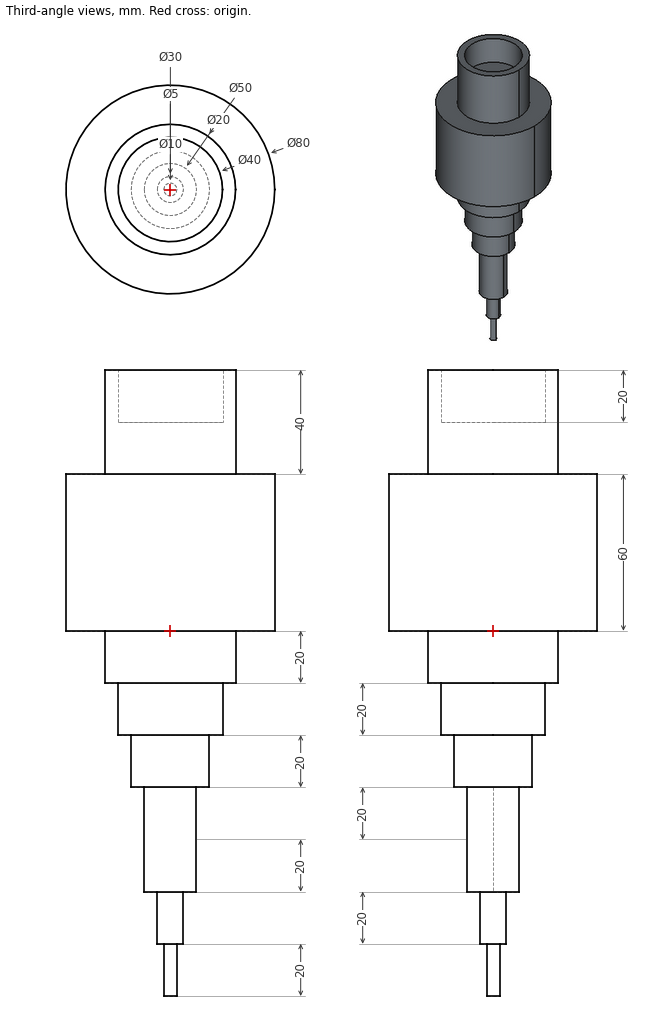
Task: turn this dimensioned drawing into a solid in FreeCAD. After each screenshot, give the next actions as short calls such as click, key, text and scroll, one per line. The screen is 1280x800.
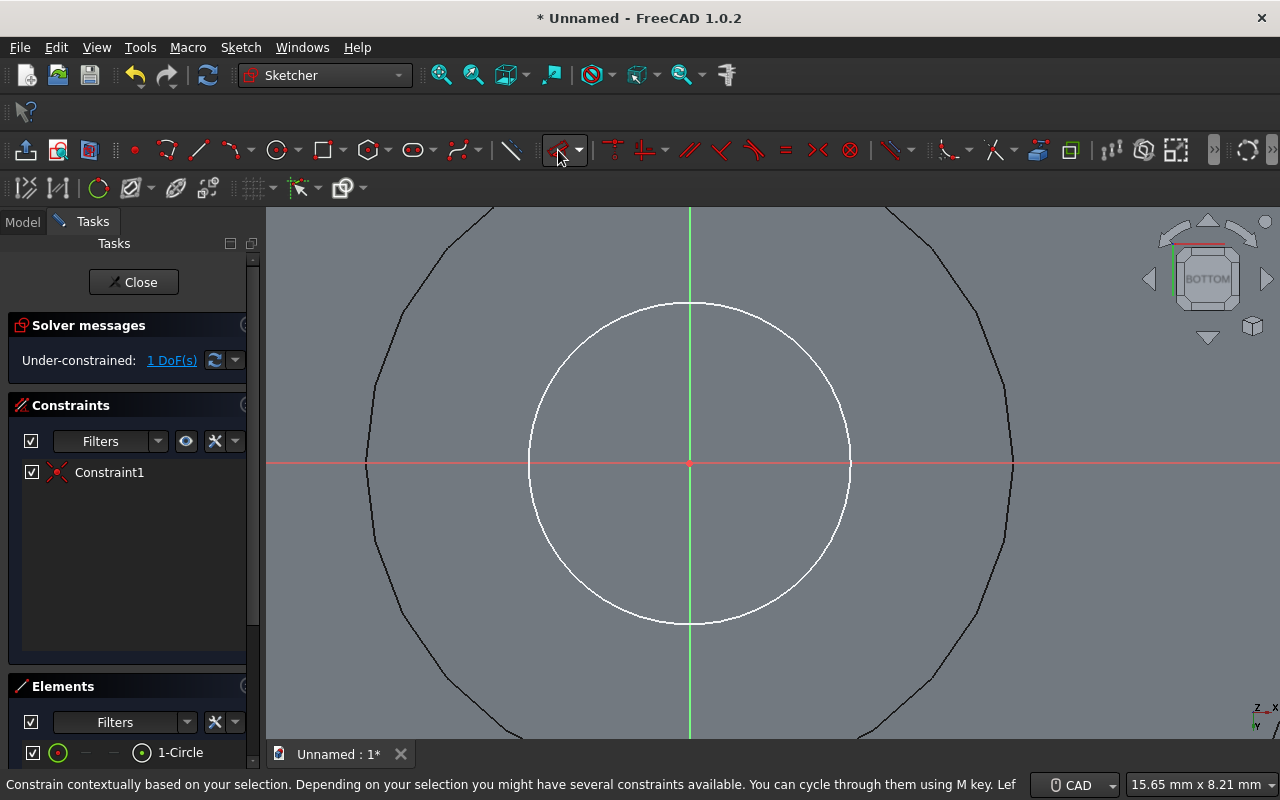
click(803, 349)
click(826, 326)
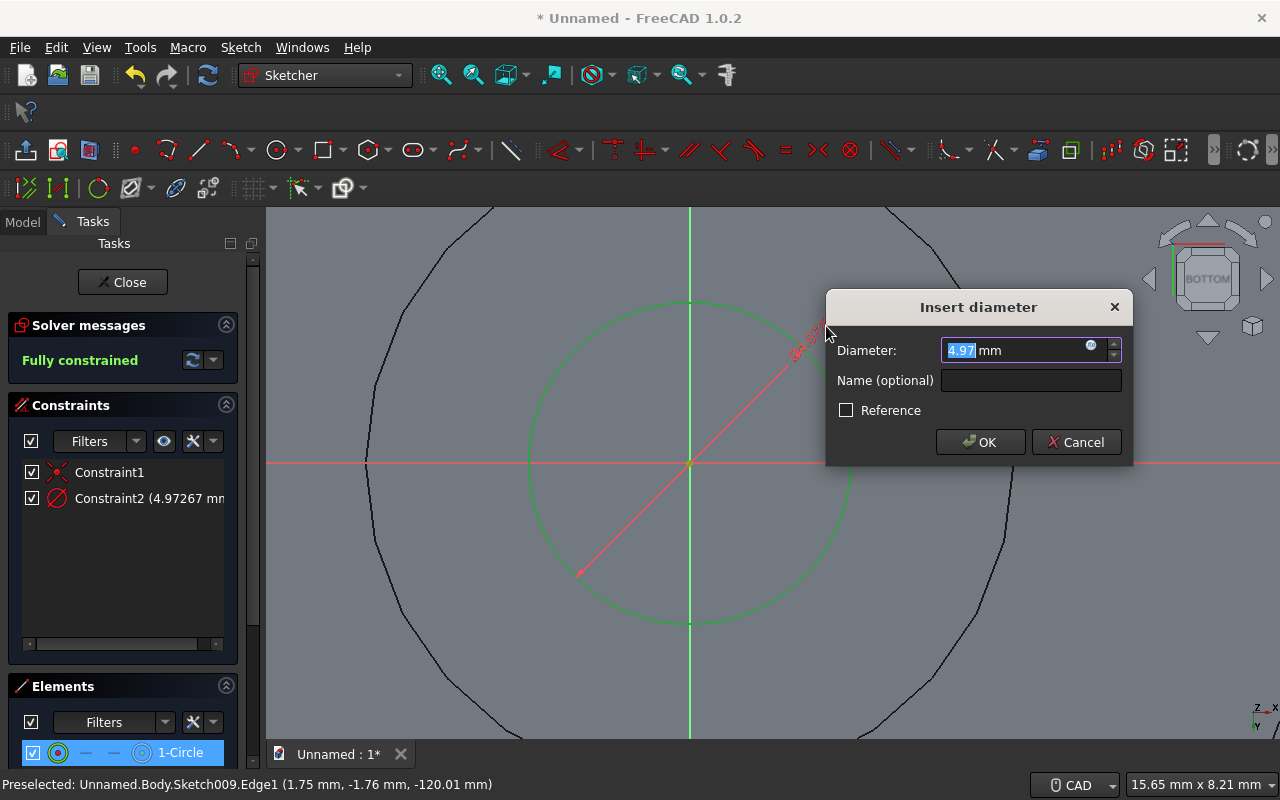
text(5)
key(Return)
key(Escape)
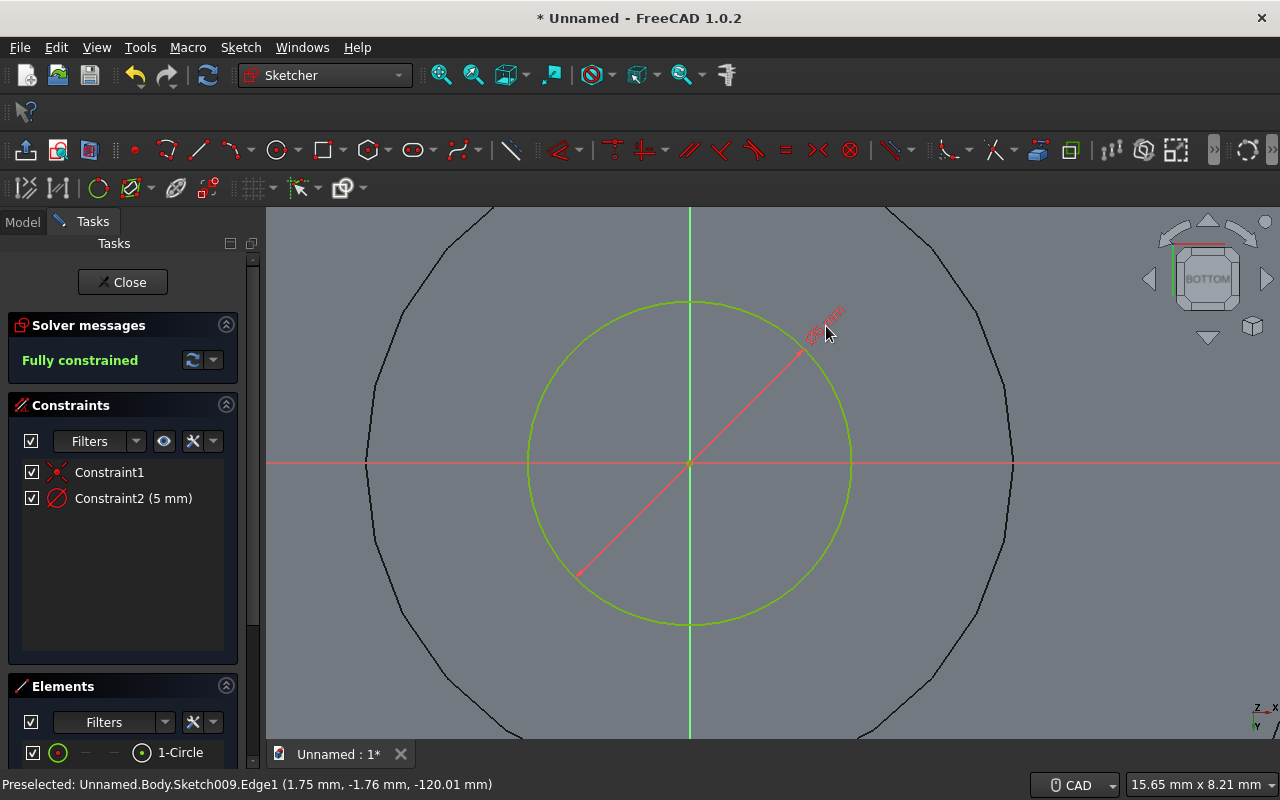
click(123, 282)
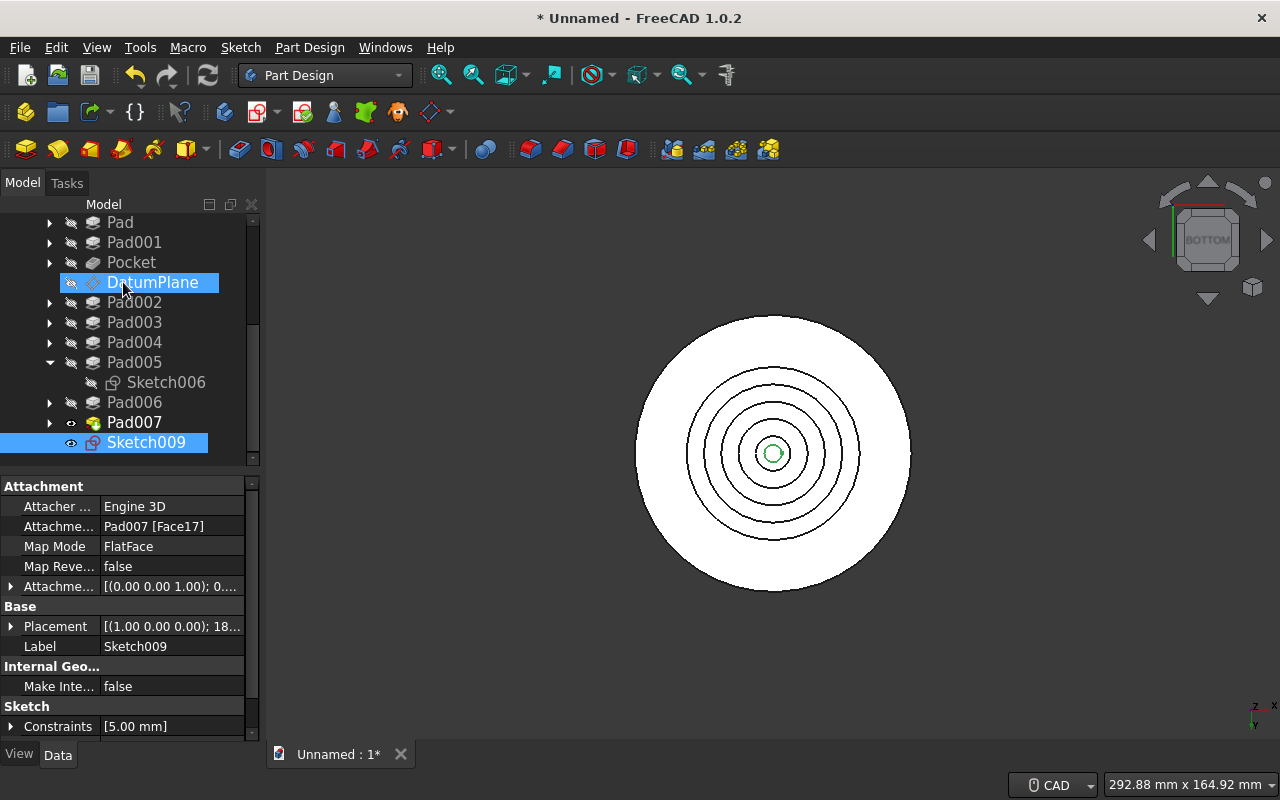
click(26, 150)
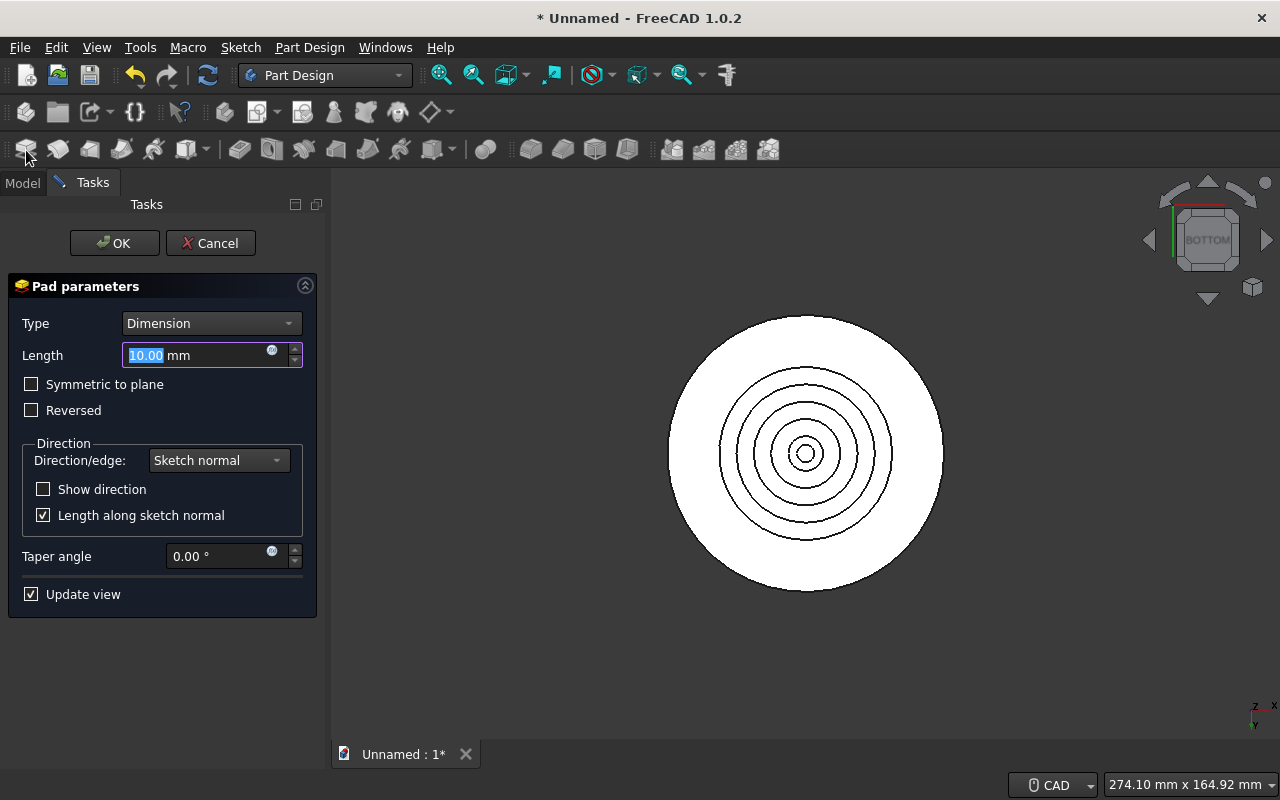
text(20)
key(Tab)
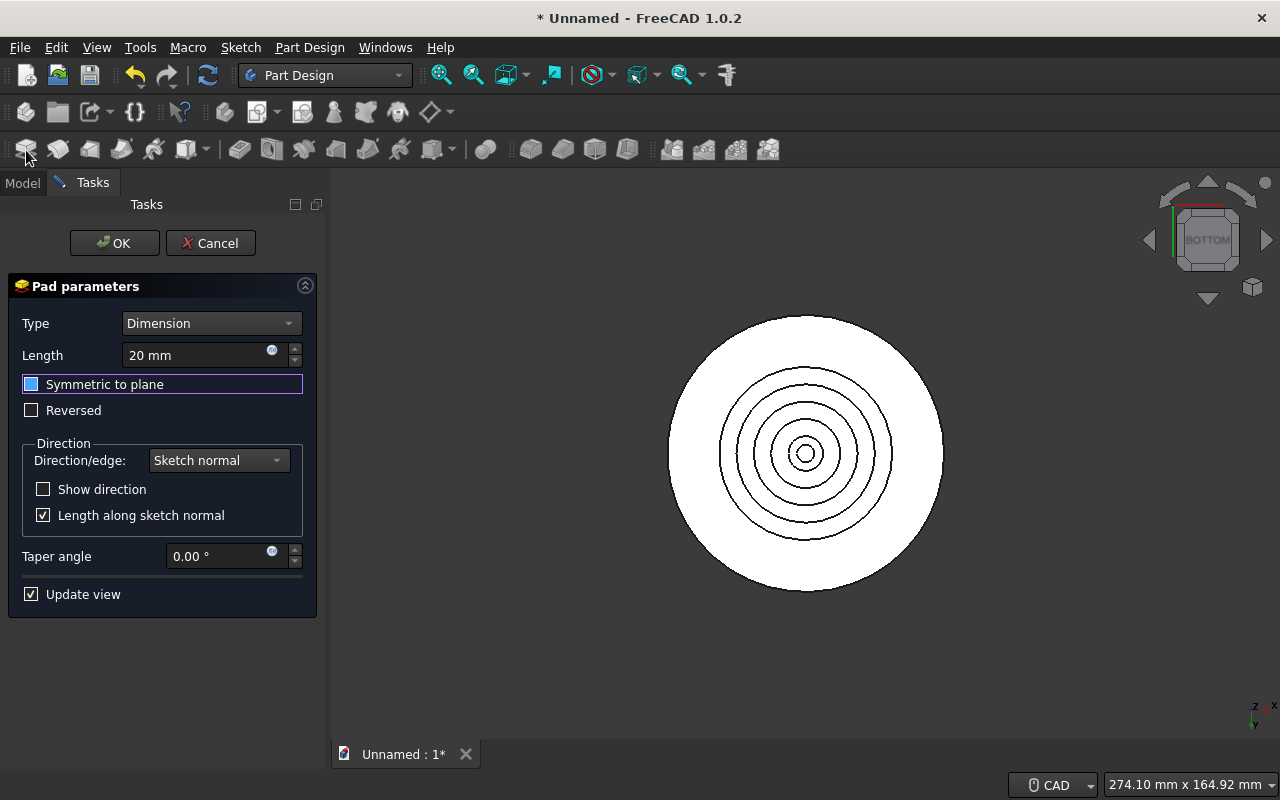
click(115, 243)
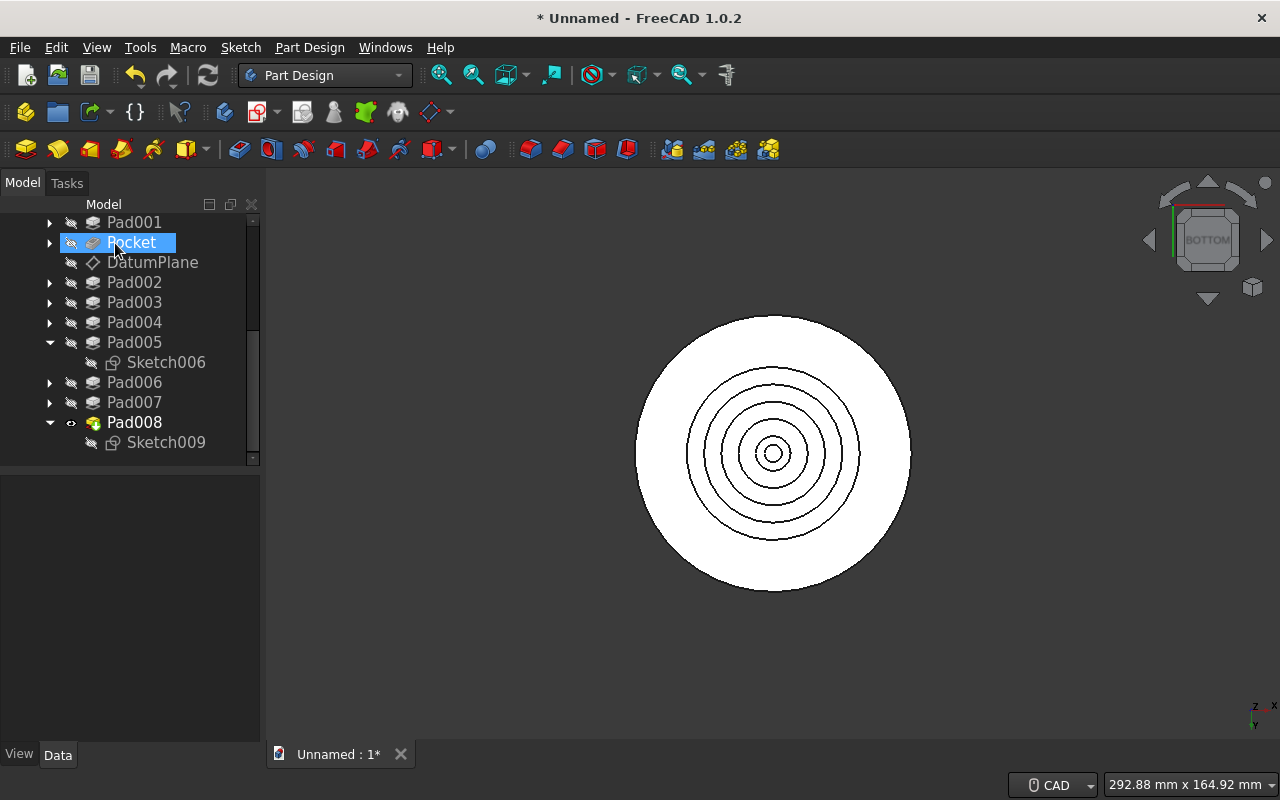
key(0)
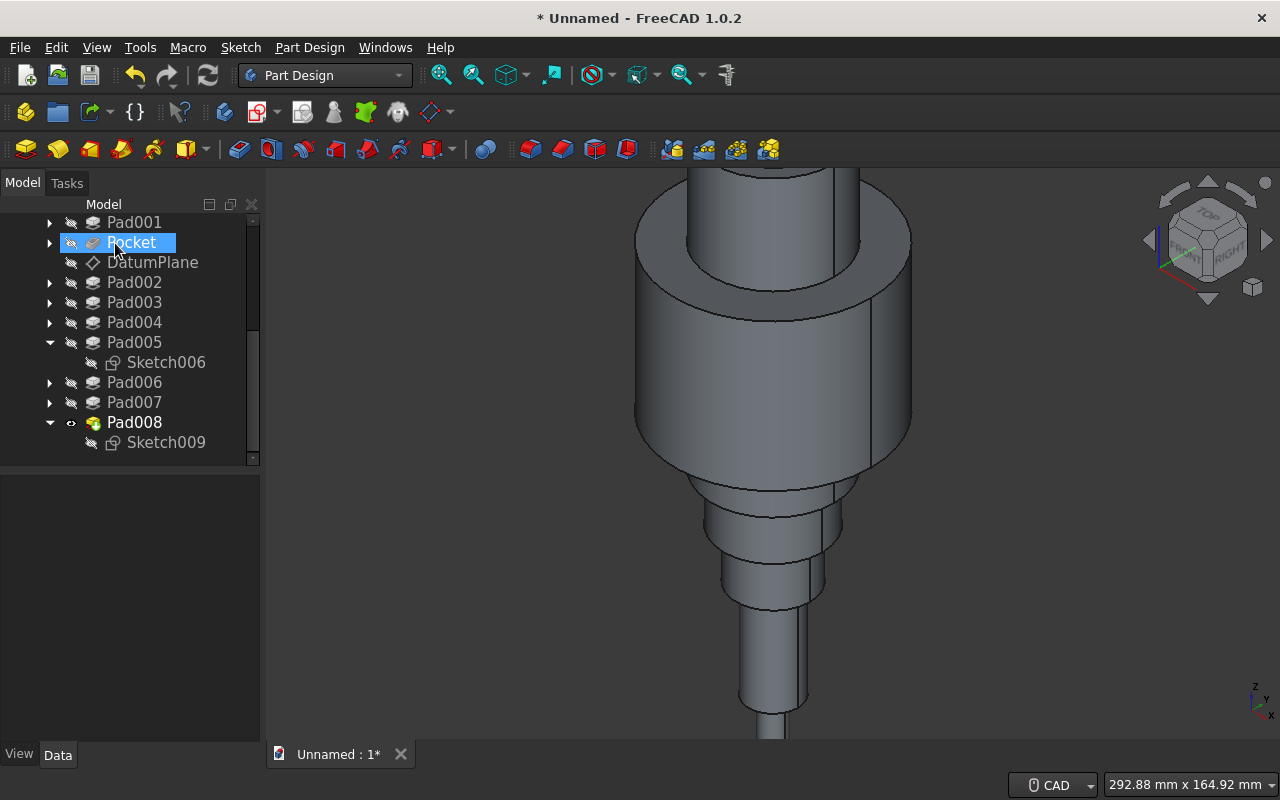
click(442, 76)